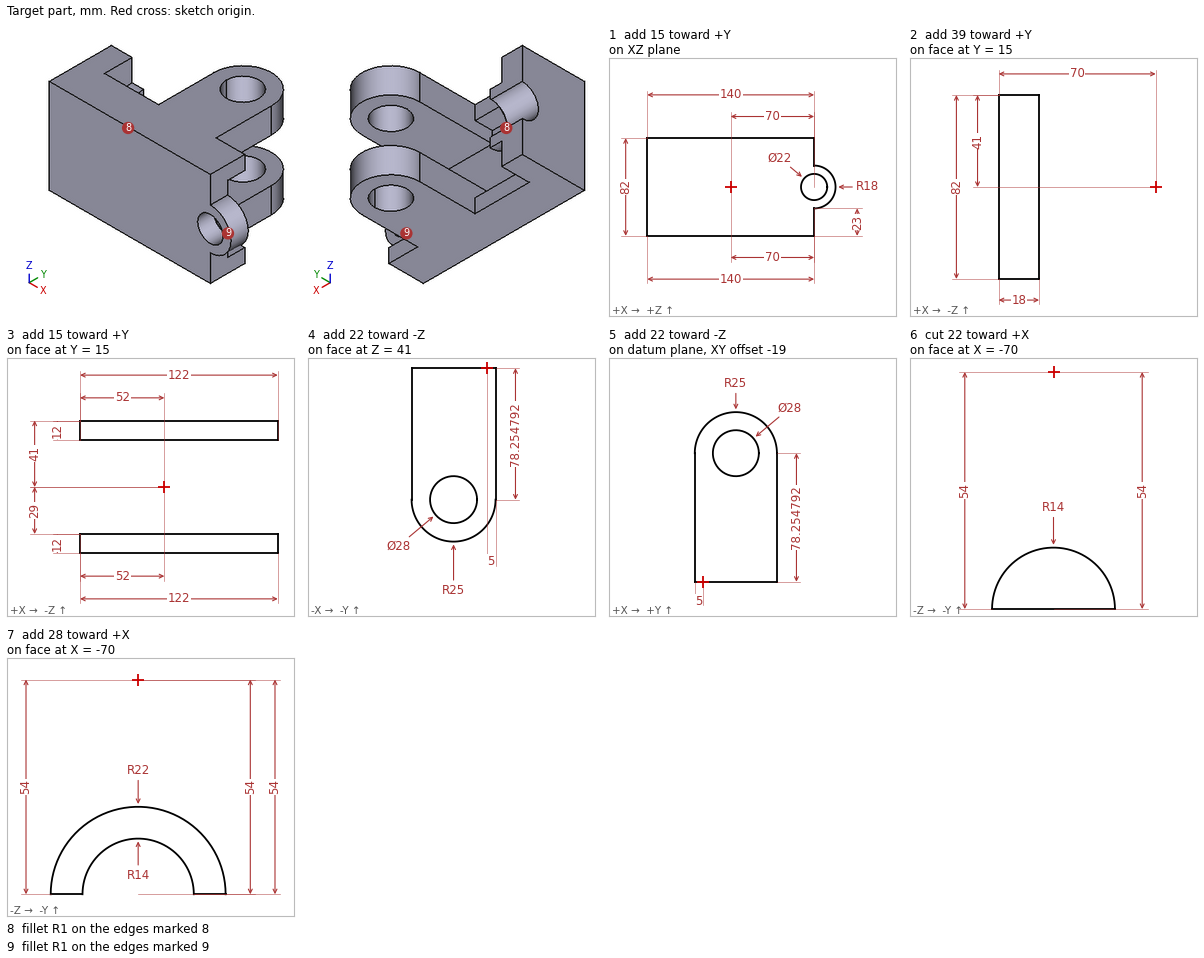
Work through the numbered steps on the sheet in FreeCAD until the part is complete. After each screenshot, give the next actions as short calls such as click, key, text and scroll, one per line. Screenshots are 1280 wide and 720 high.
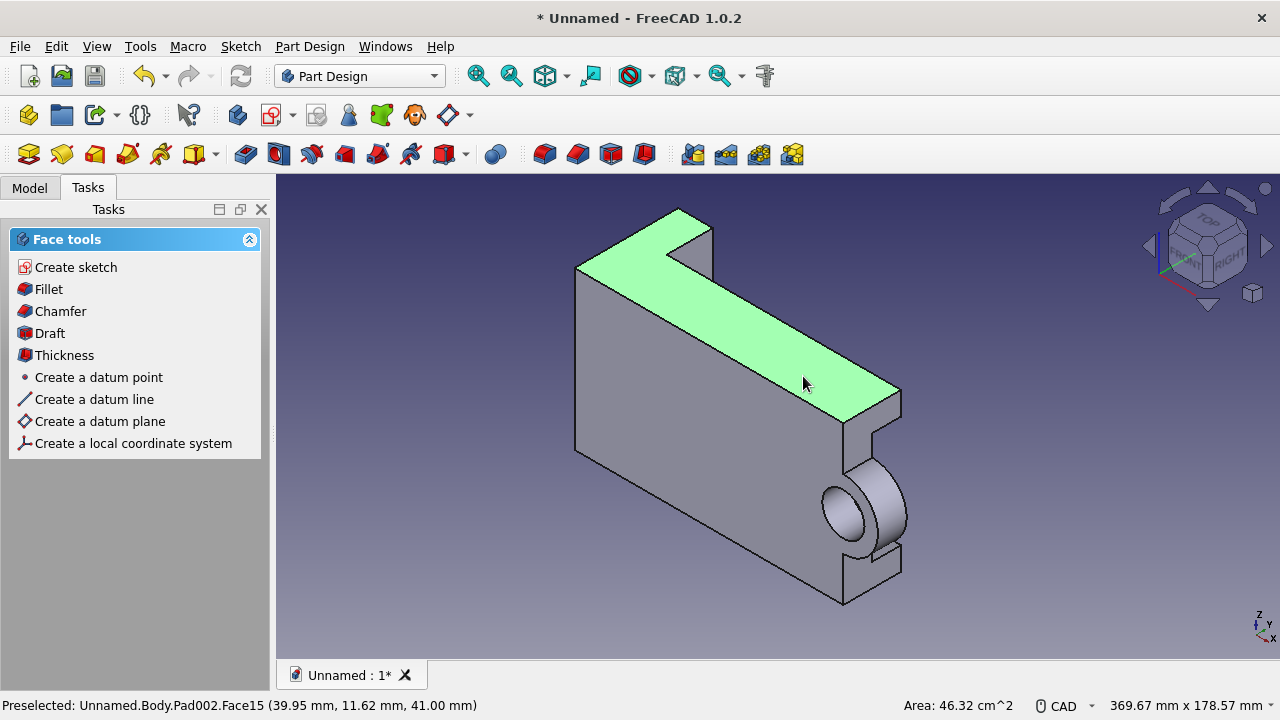
click(270, 116)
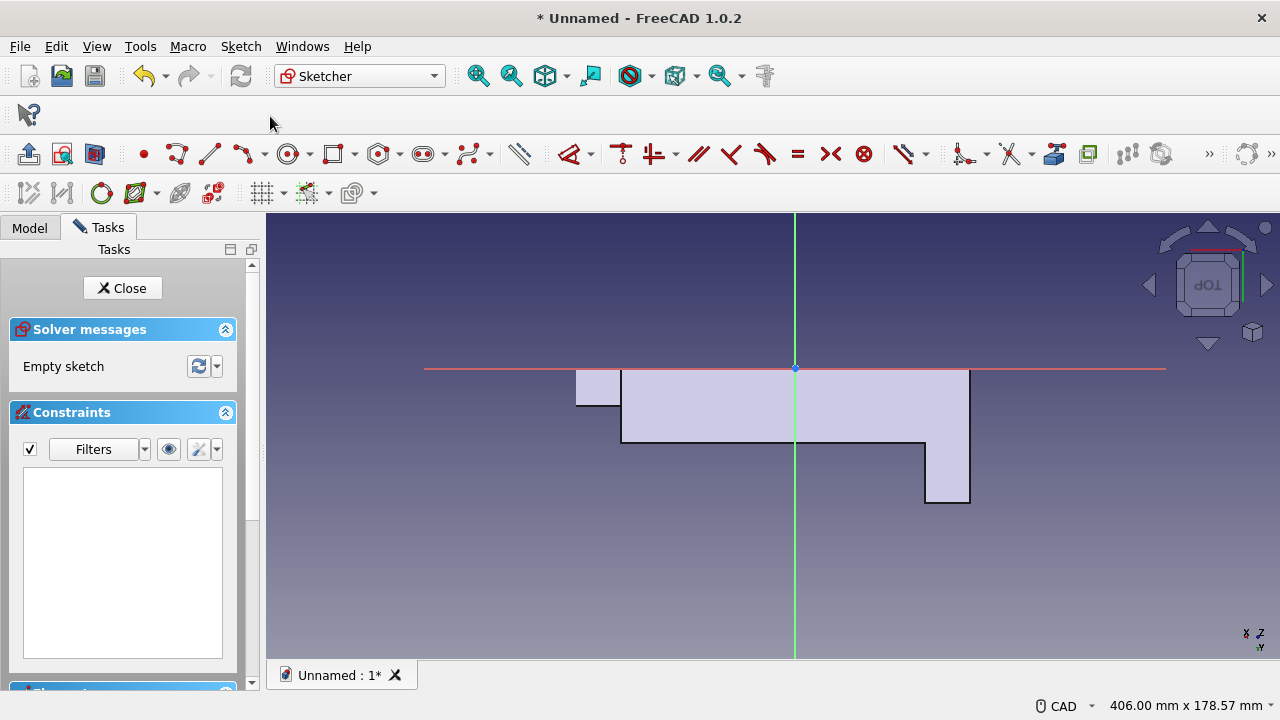
scroll(520, 241, down, 1)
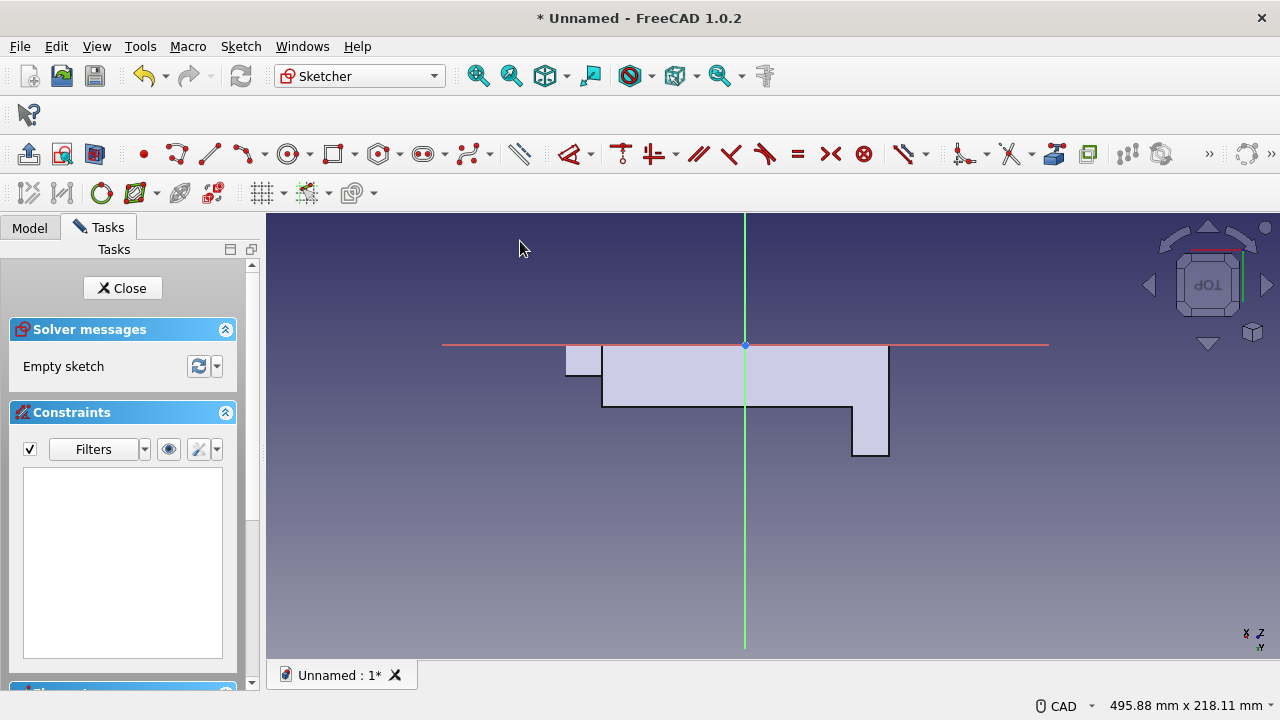
click(177, 154)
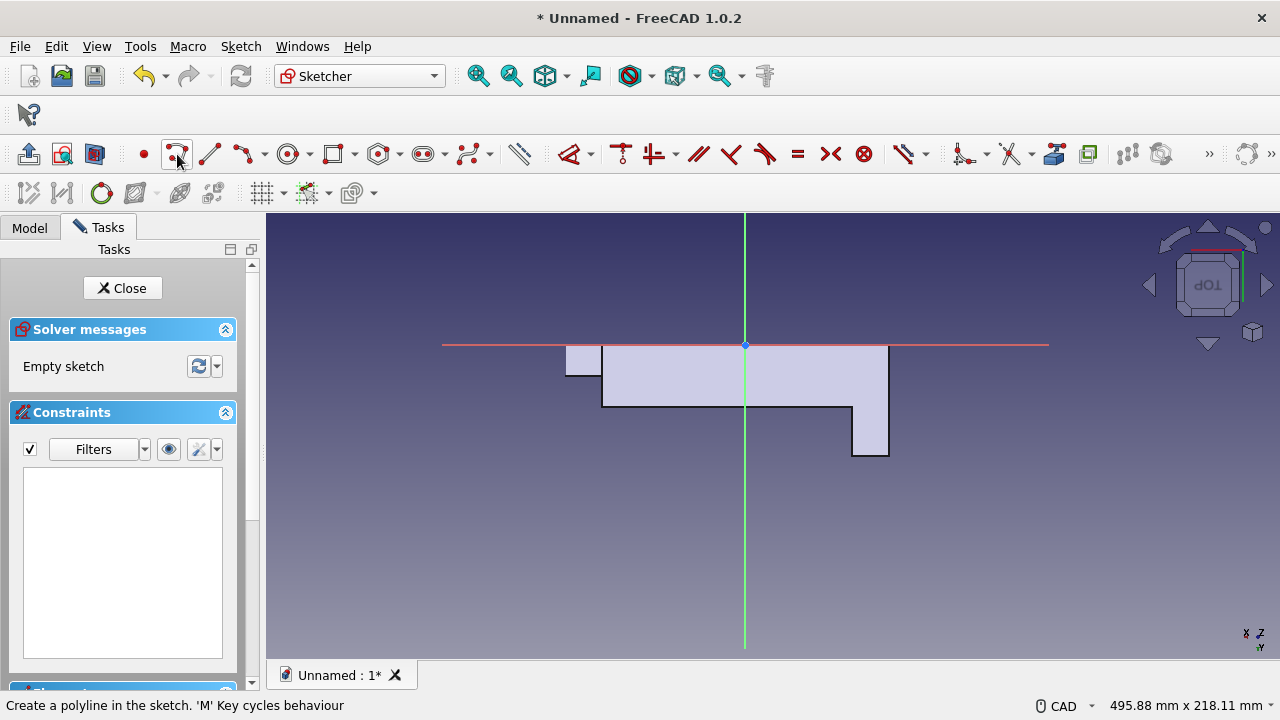
scroll(756, 505, up, 3)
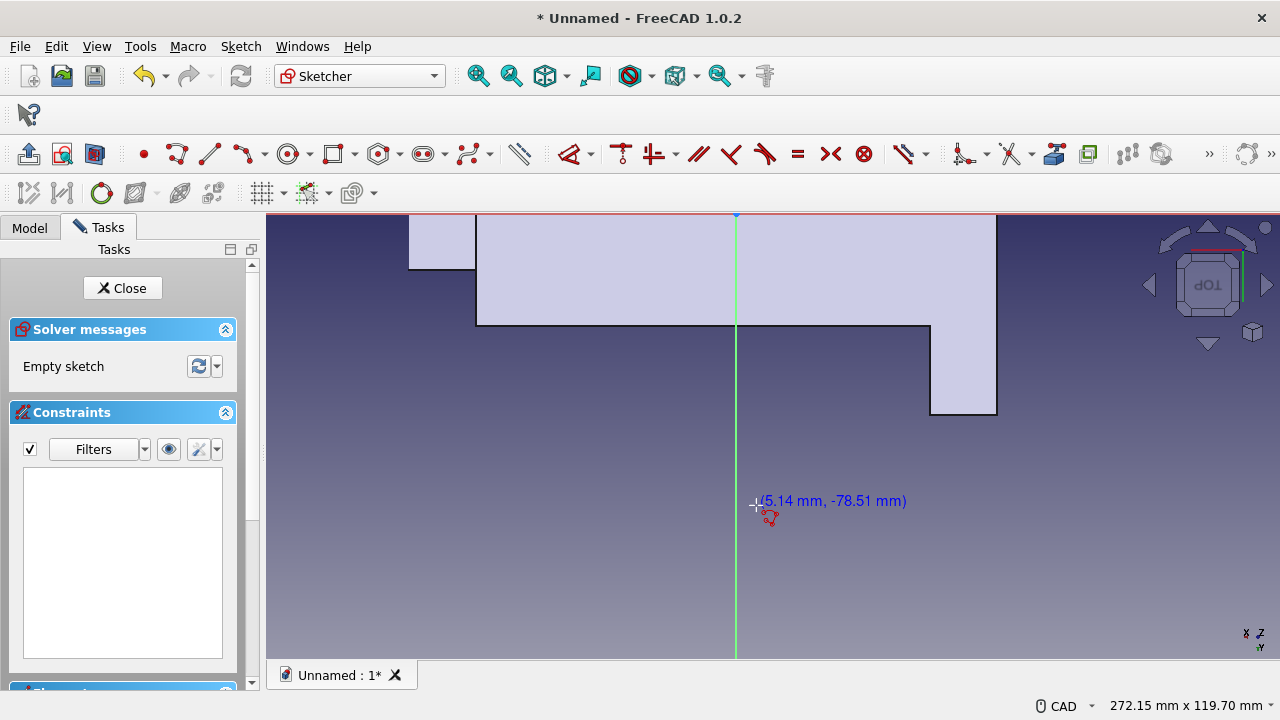
click(755, 505)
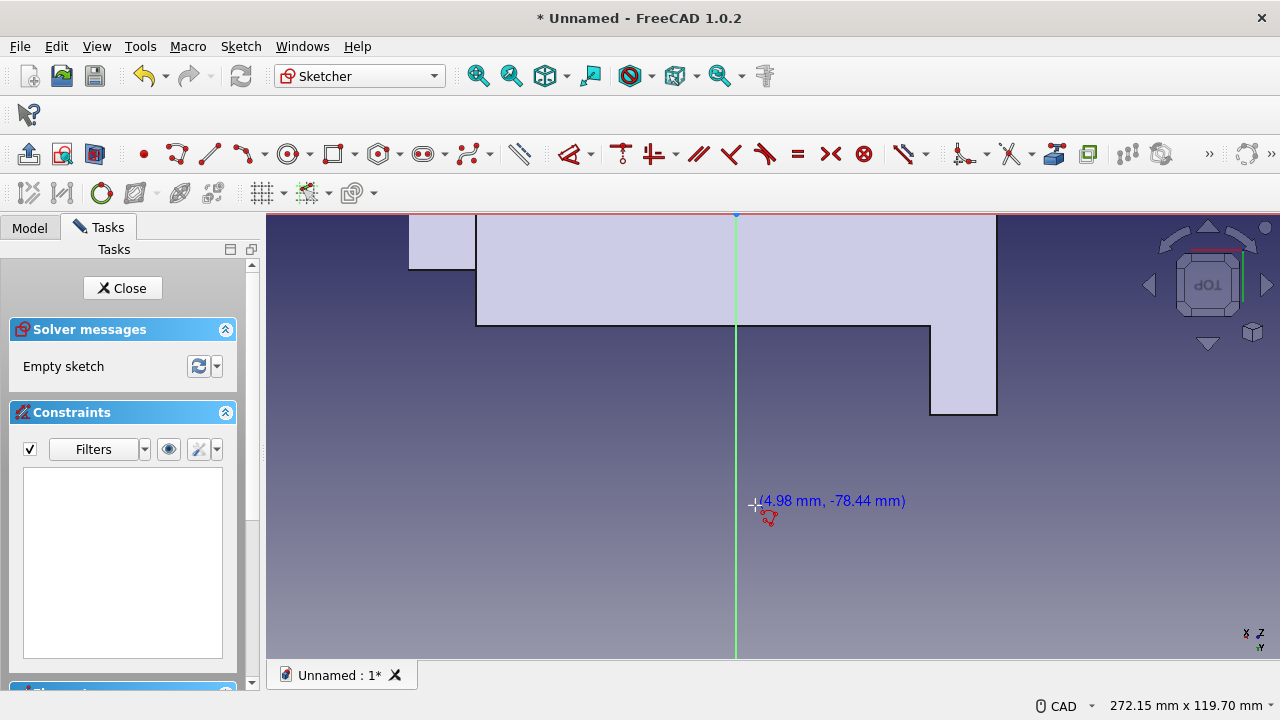
scroll(791, 497, down, 2)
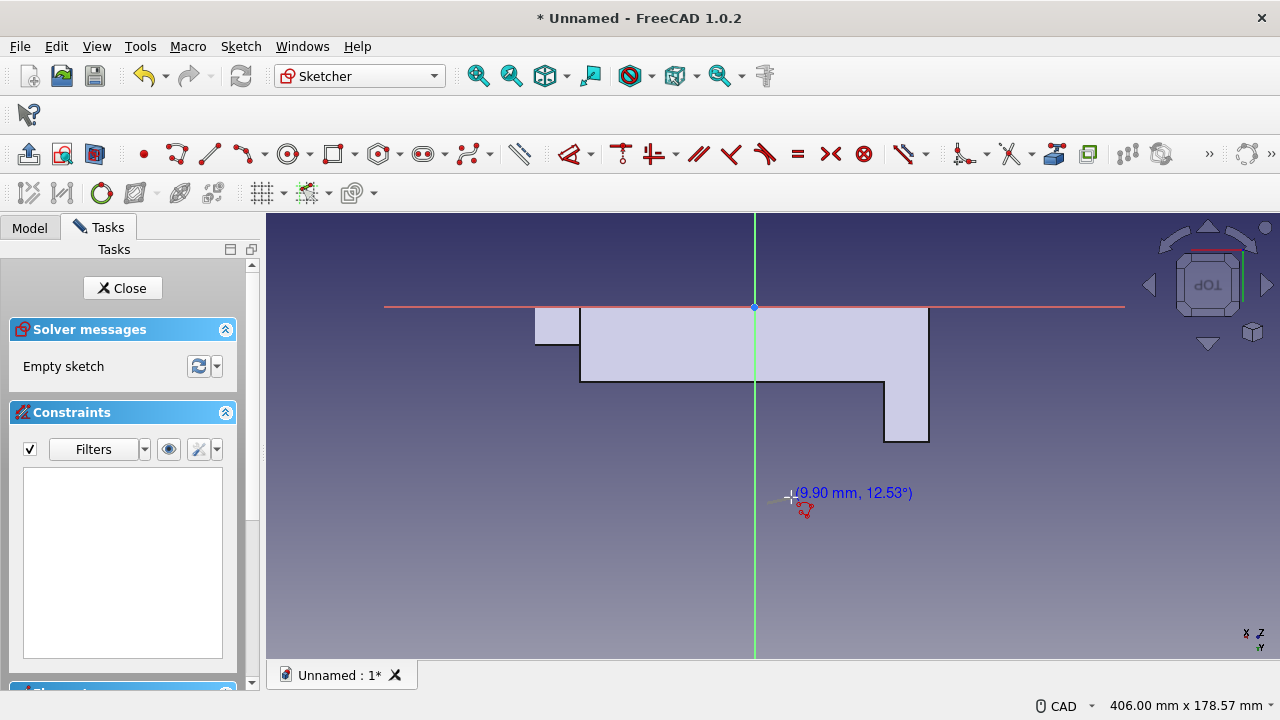
scroll(767, 307, up, 2)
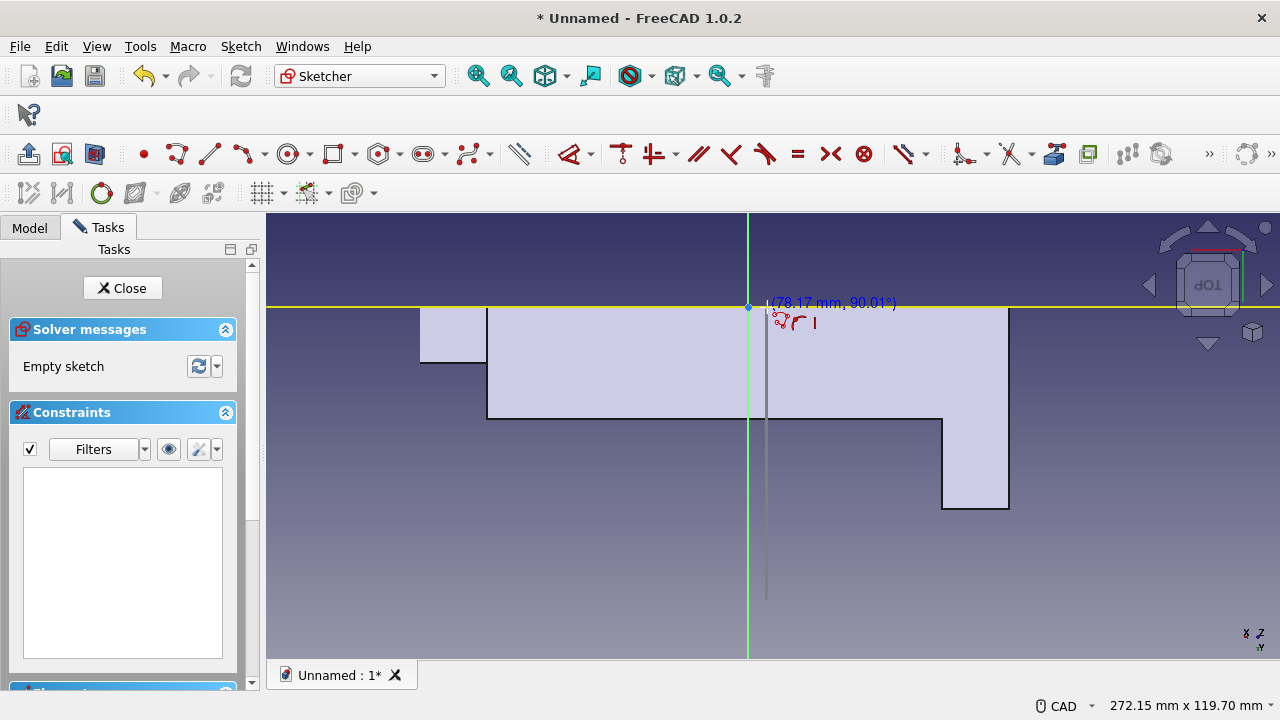
click(767, 307)
click(581, 316)
click(581, 599)
right_click(581, 599)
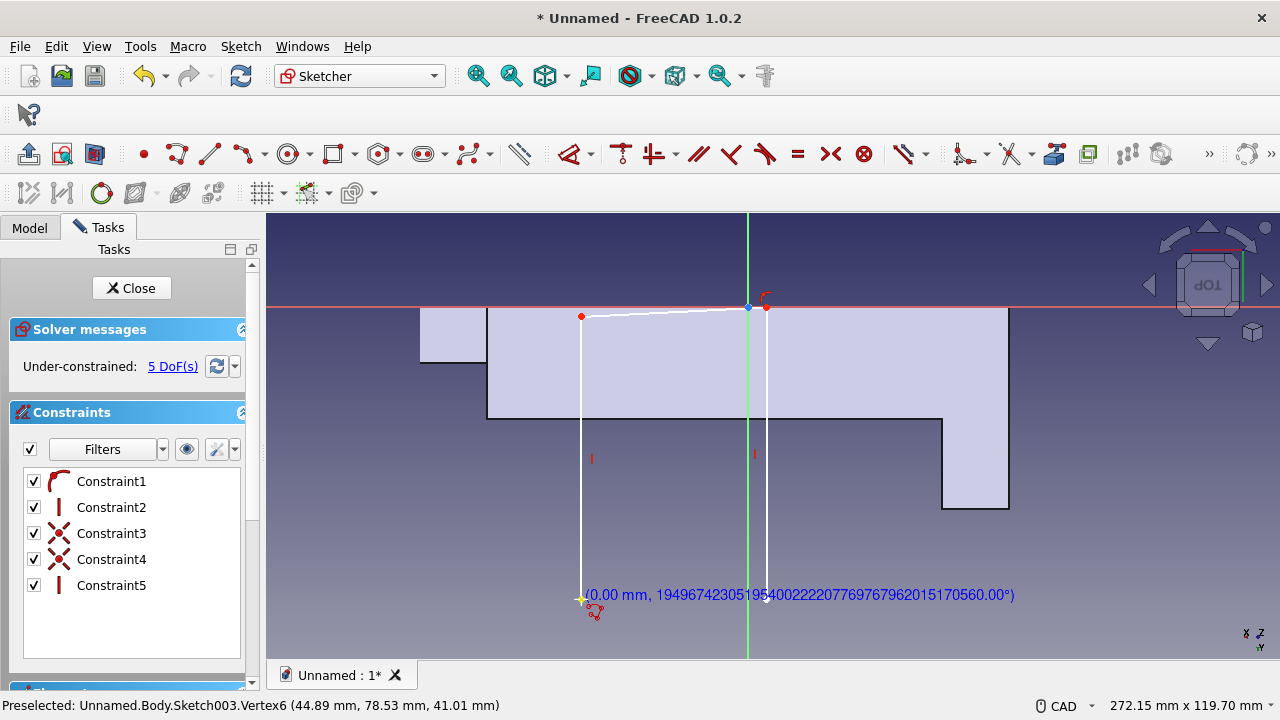
click(242, 154)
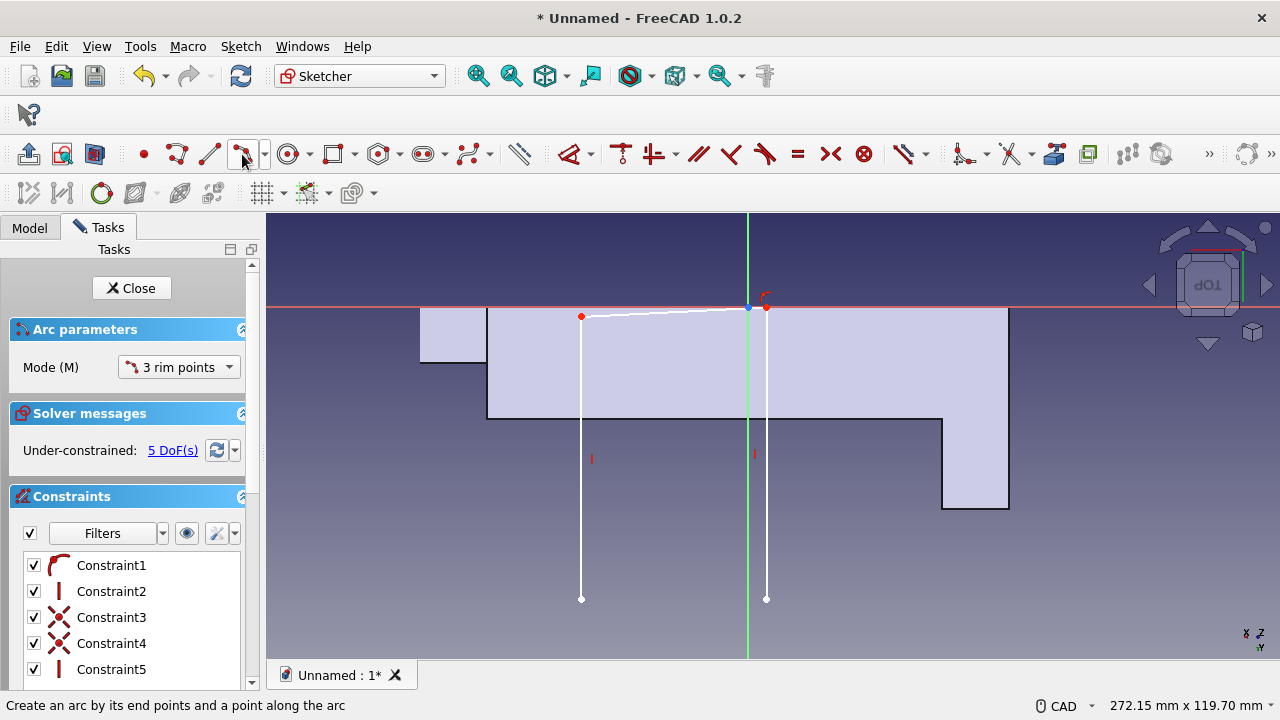
click(581, 600)
click(767, 600)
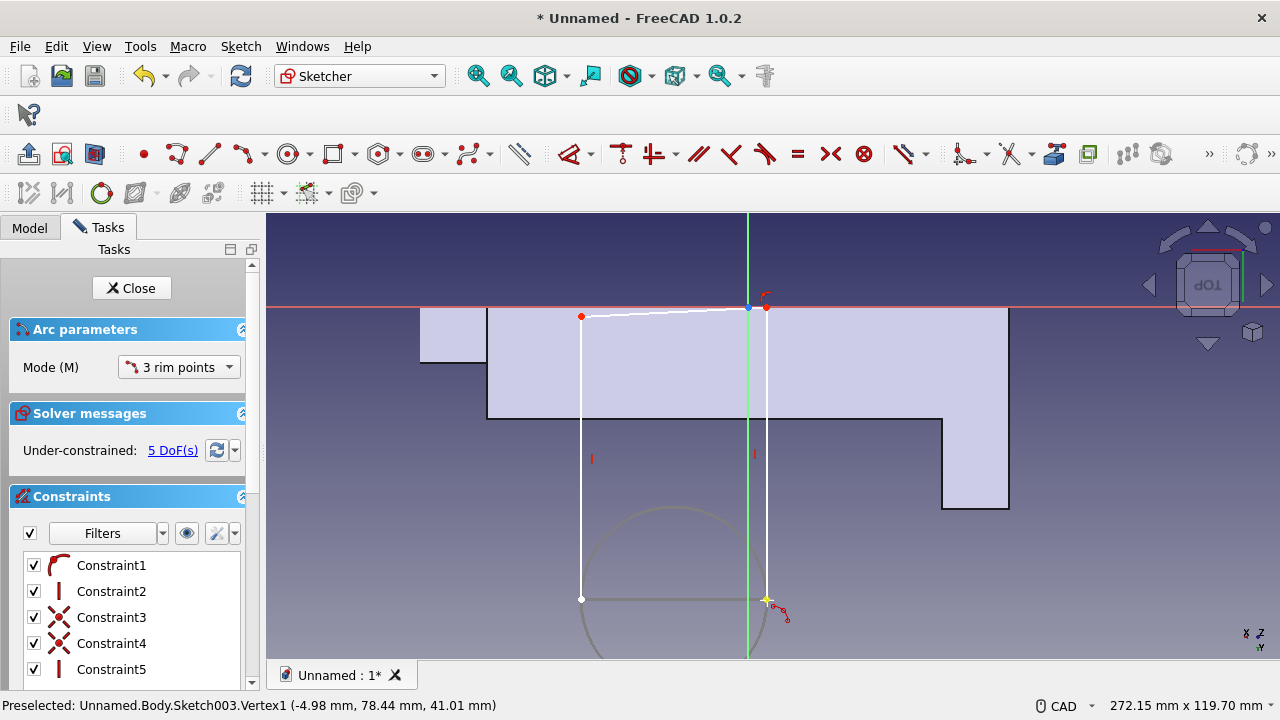
scroll(767, 306, down, 2)